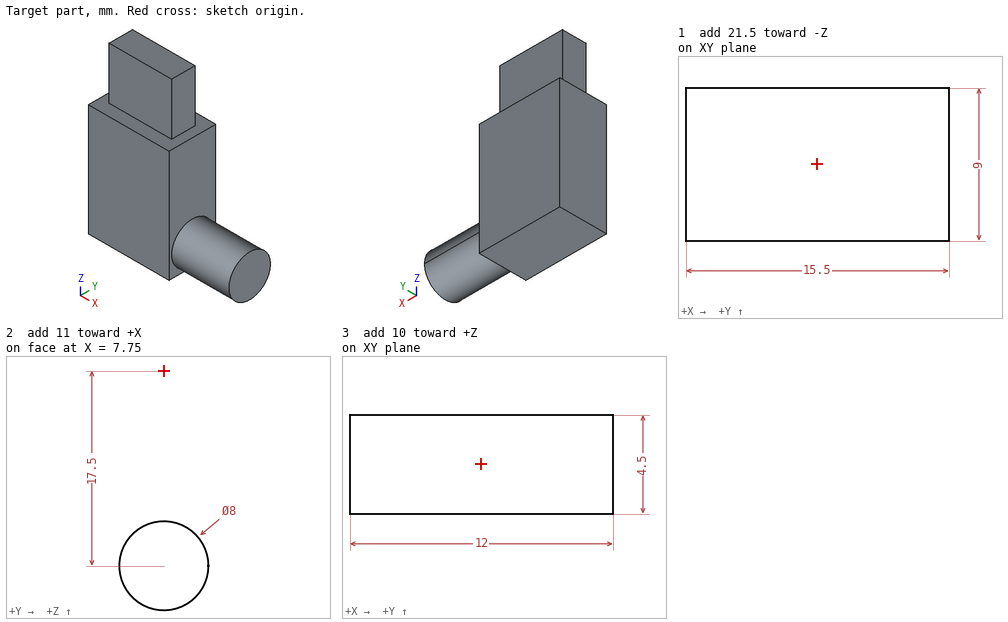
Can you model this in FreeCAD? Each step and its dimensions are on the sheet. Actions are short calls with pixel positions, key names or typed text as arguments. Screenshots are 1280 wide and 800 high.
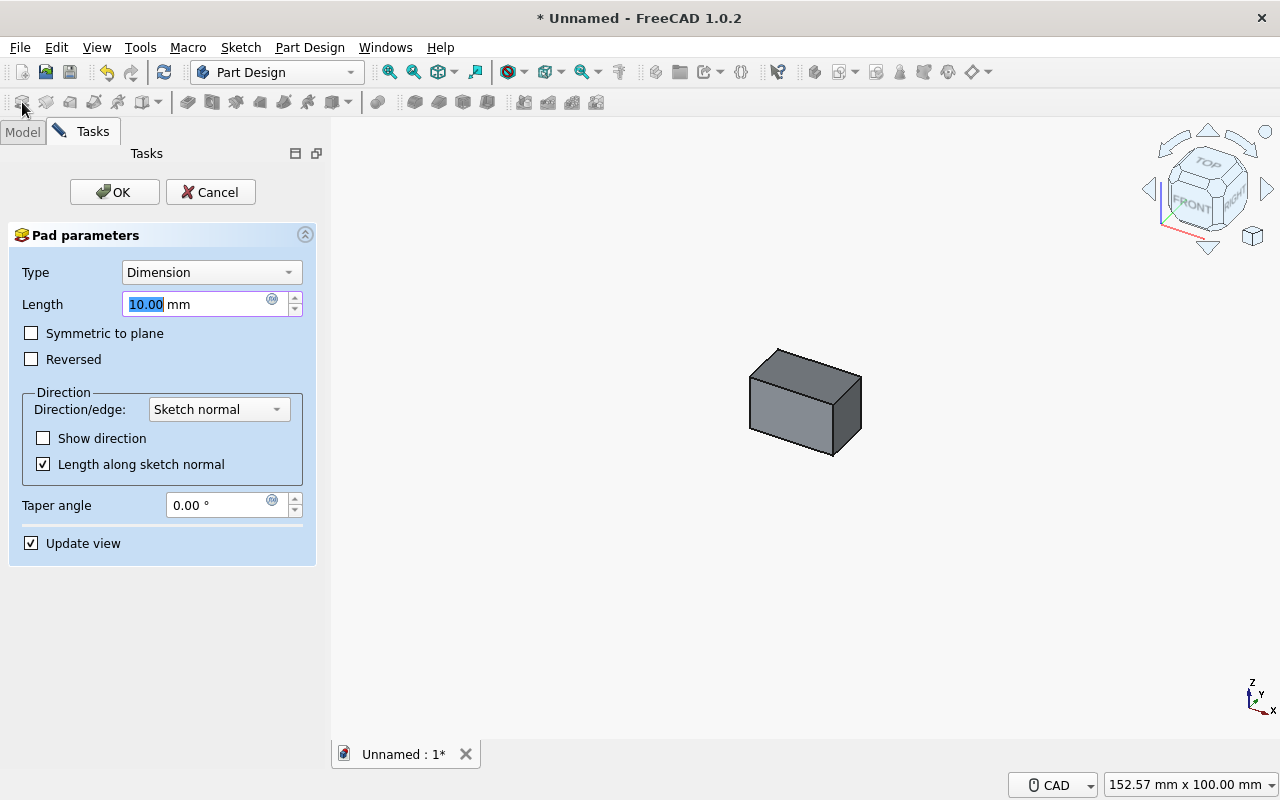
text(21.5)
key(Tab)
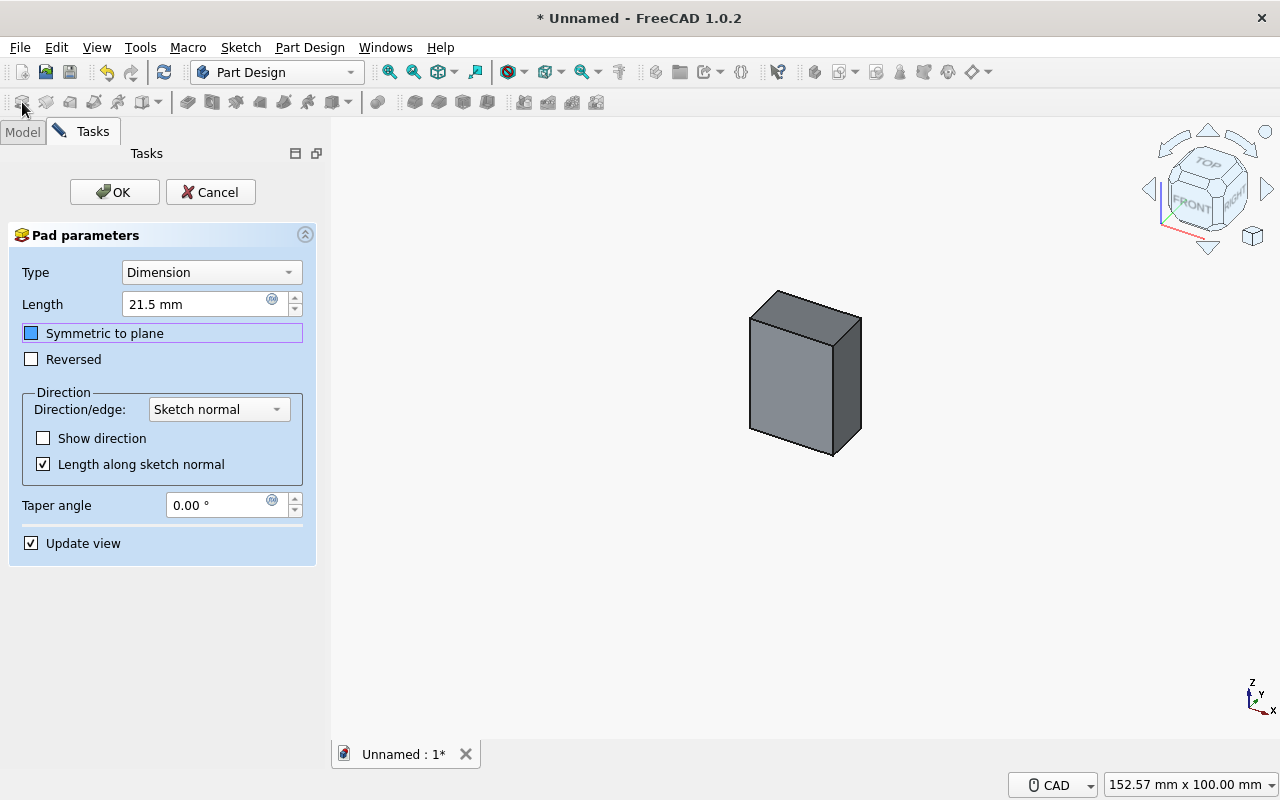
click(30, 359)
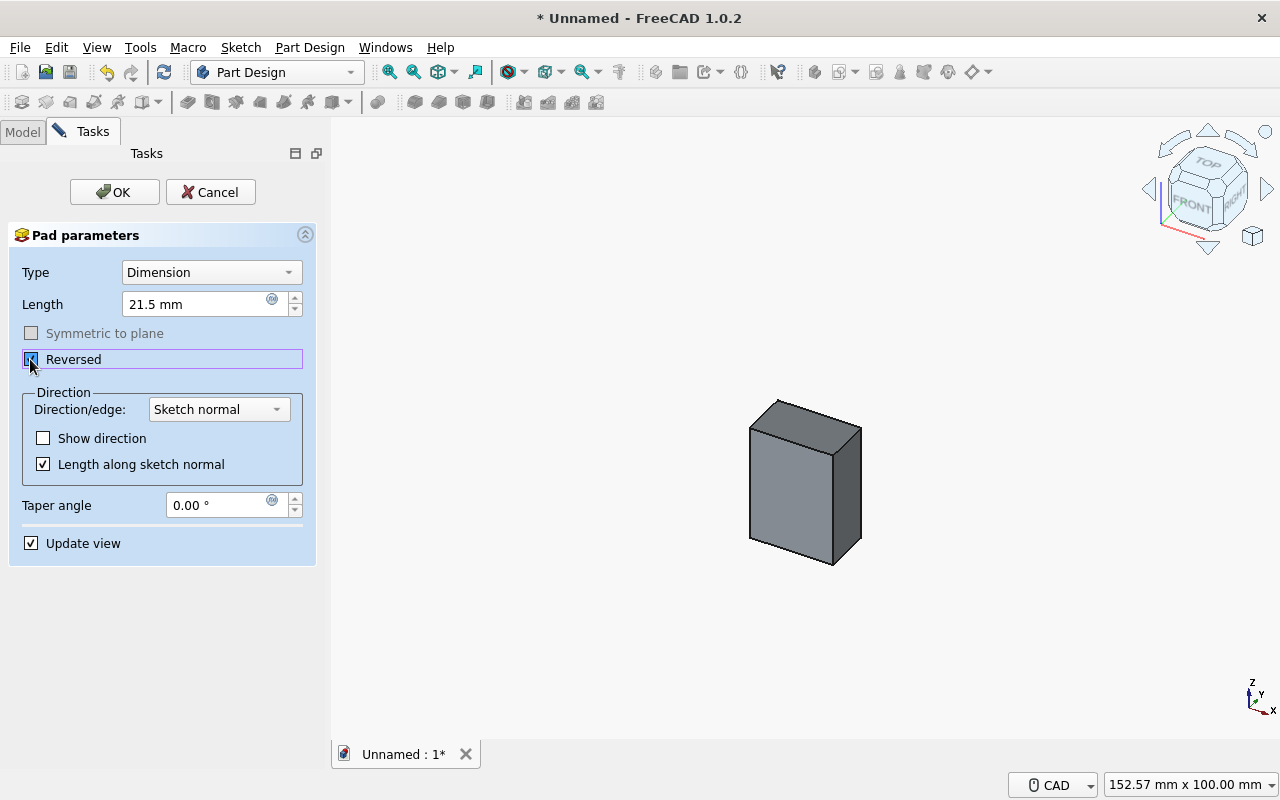
click(115, 192)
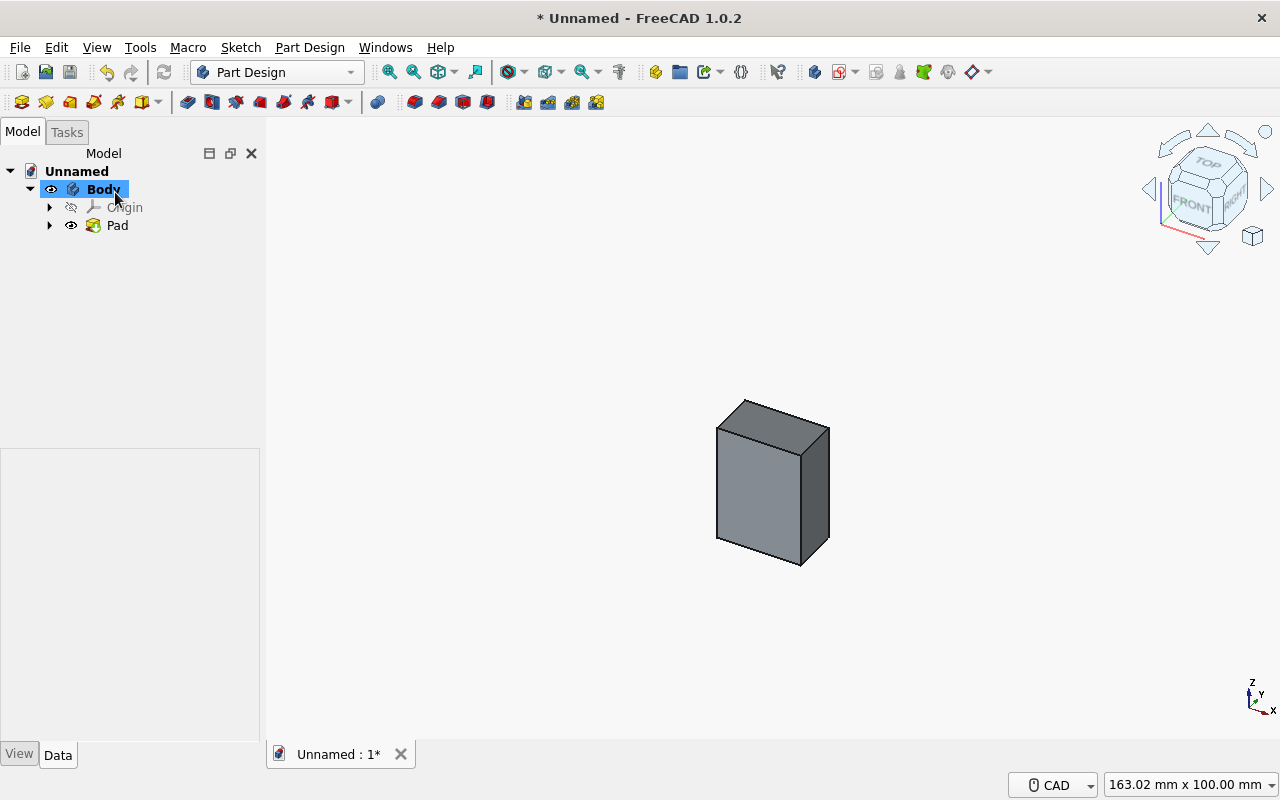
click(390, 72)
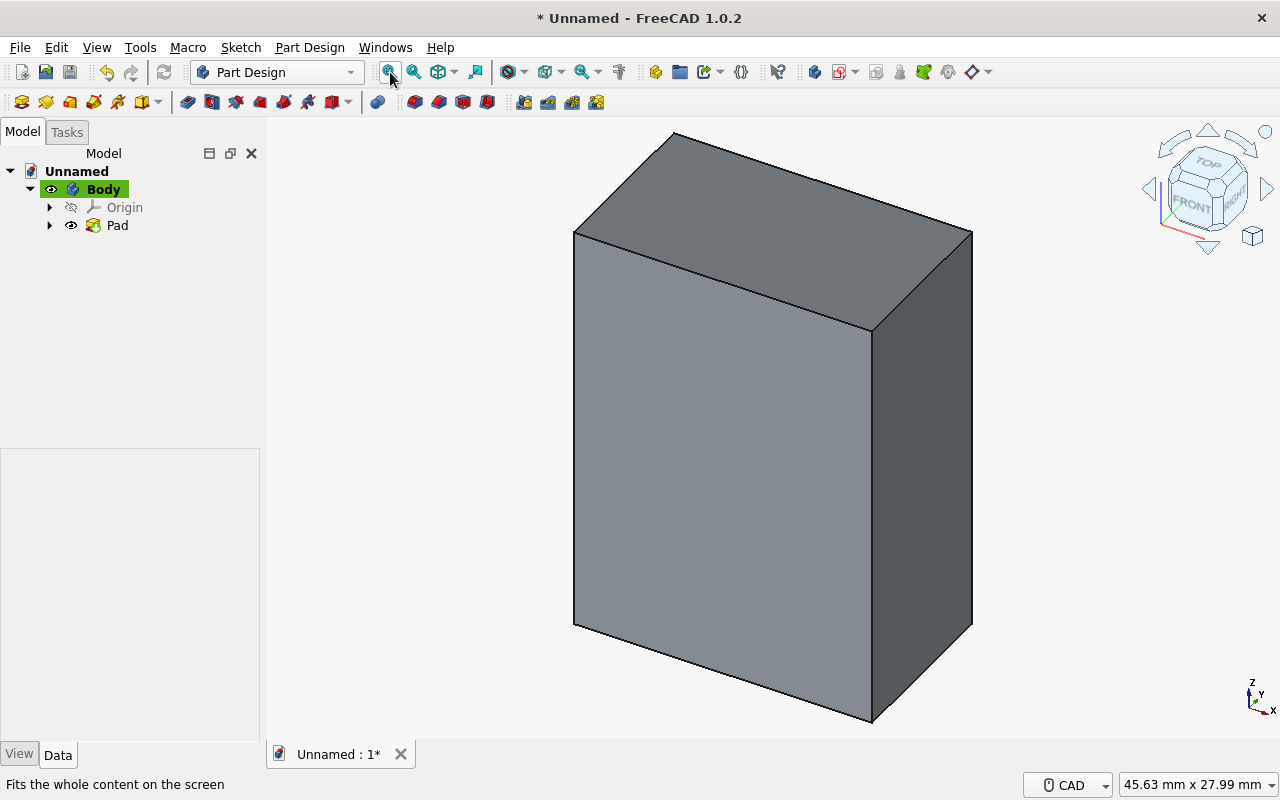
click(922, 365)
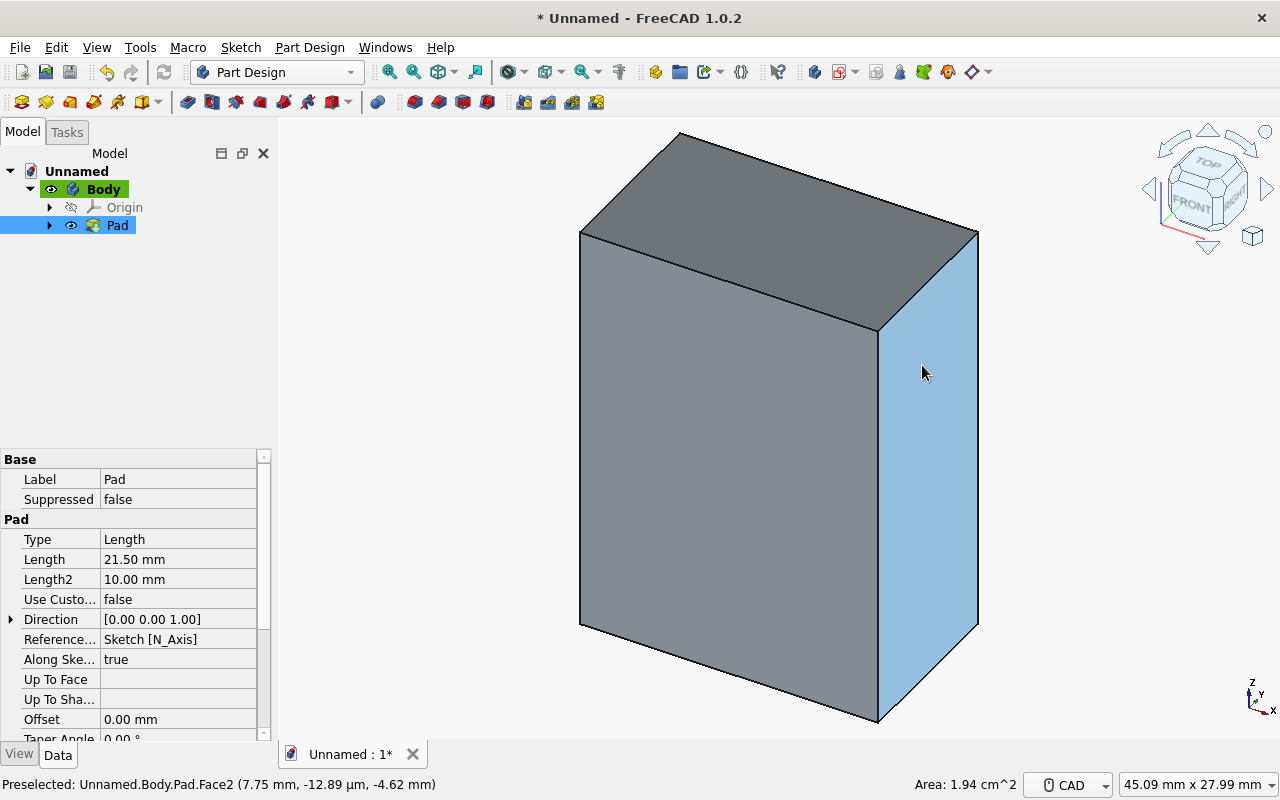
click(840, 72)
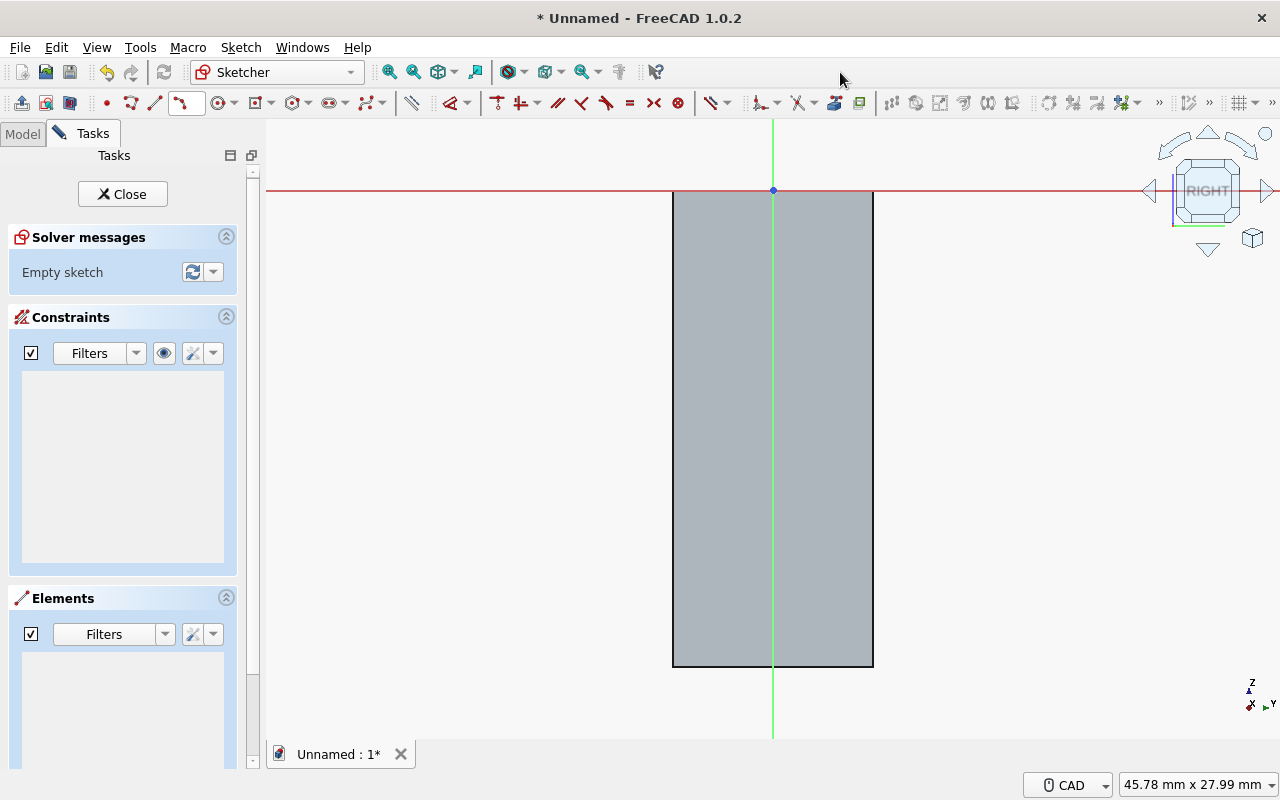
scroll(829, 701, up, 4)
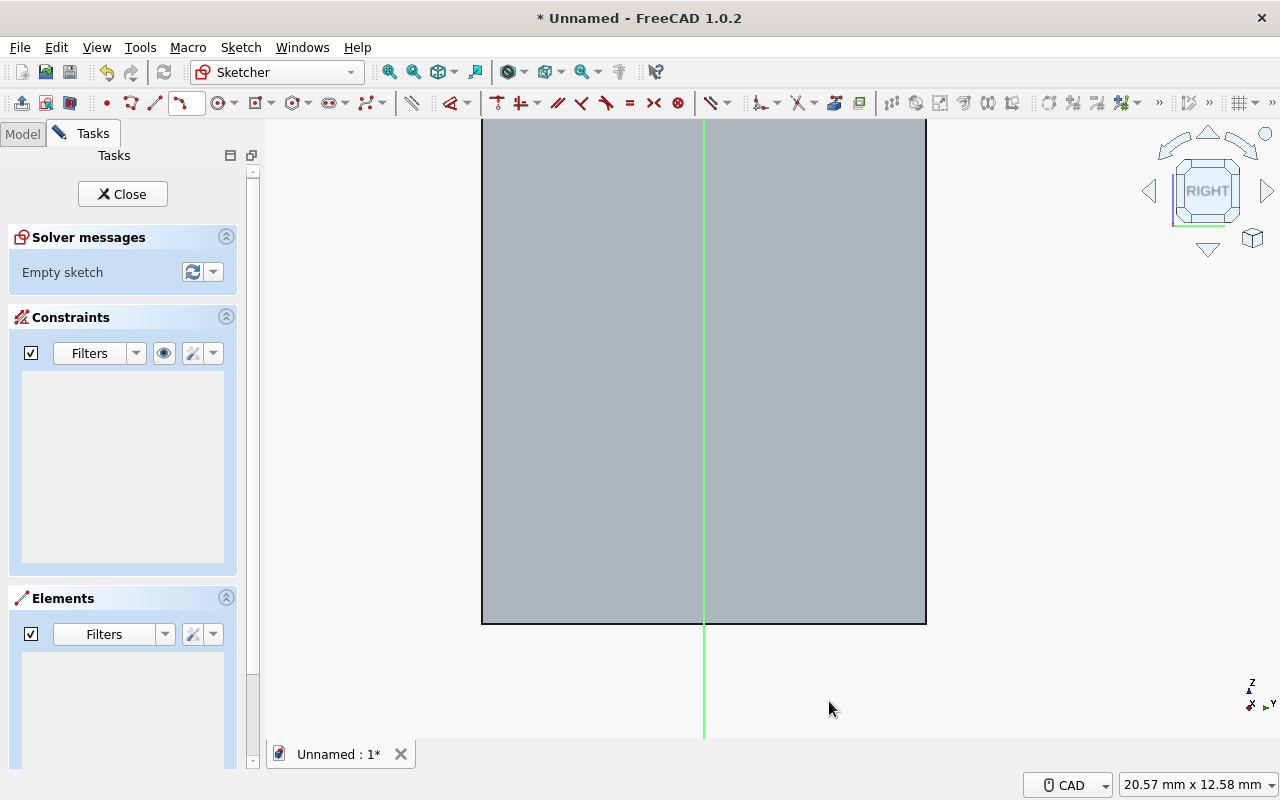
click(218, 104)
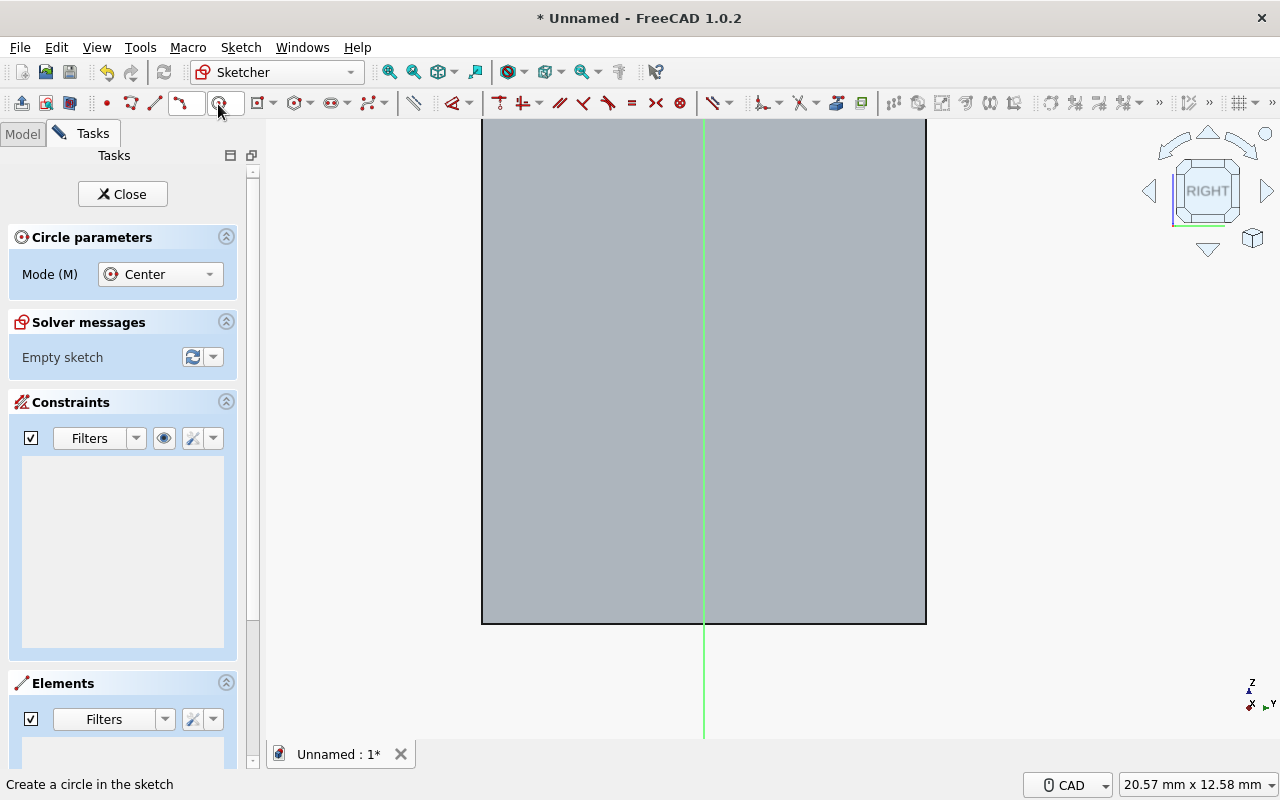
click(704, 427)
move(843, 288)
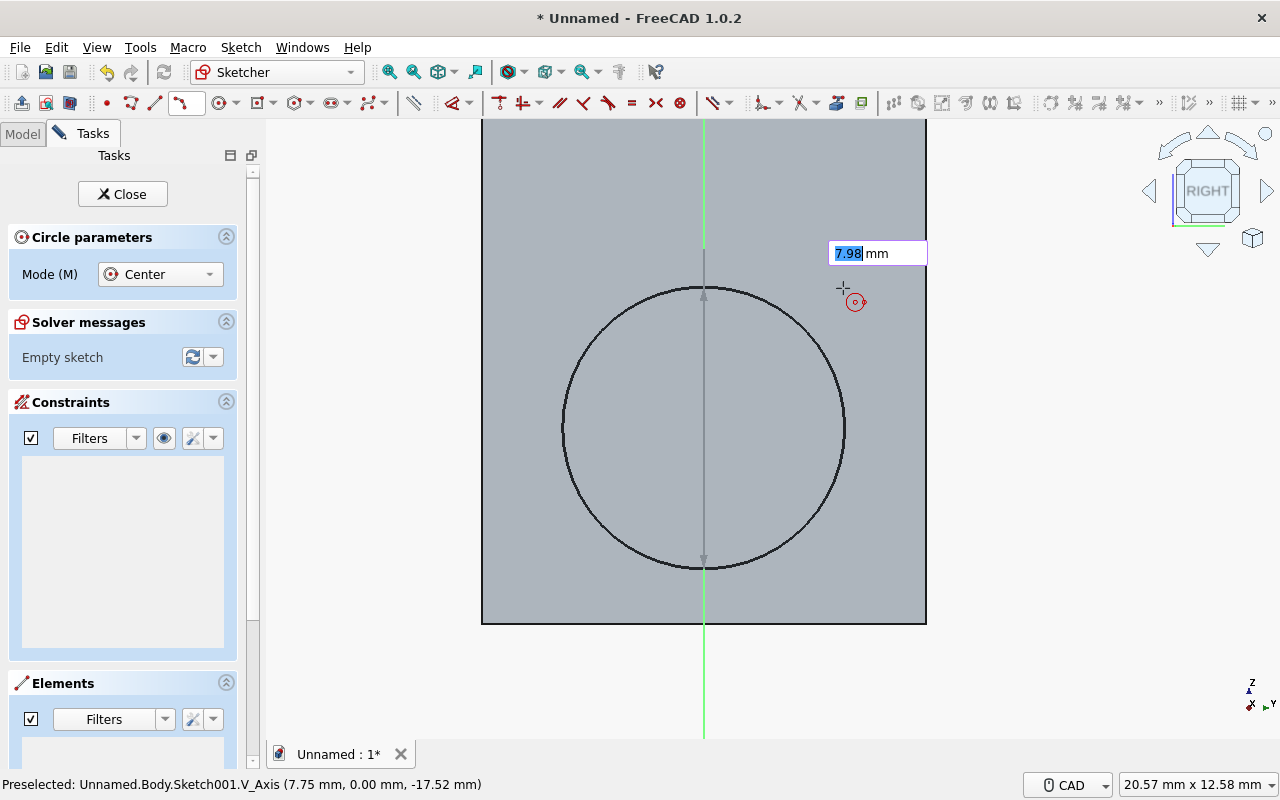
text(8)
key(Return)
key(Escape)